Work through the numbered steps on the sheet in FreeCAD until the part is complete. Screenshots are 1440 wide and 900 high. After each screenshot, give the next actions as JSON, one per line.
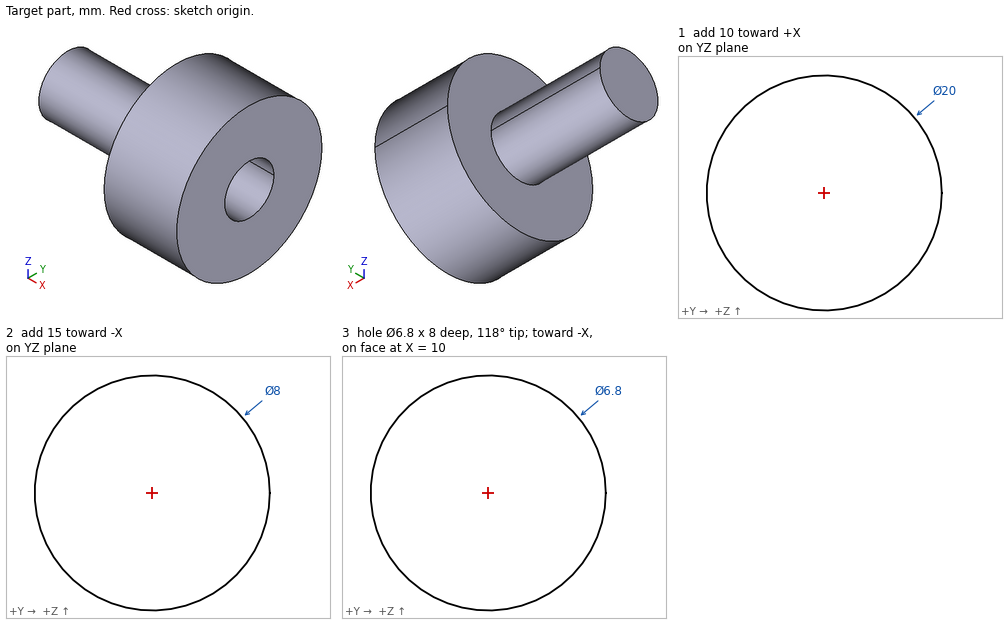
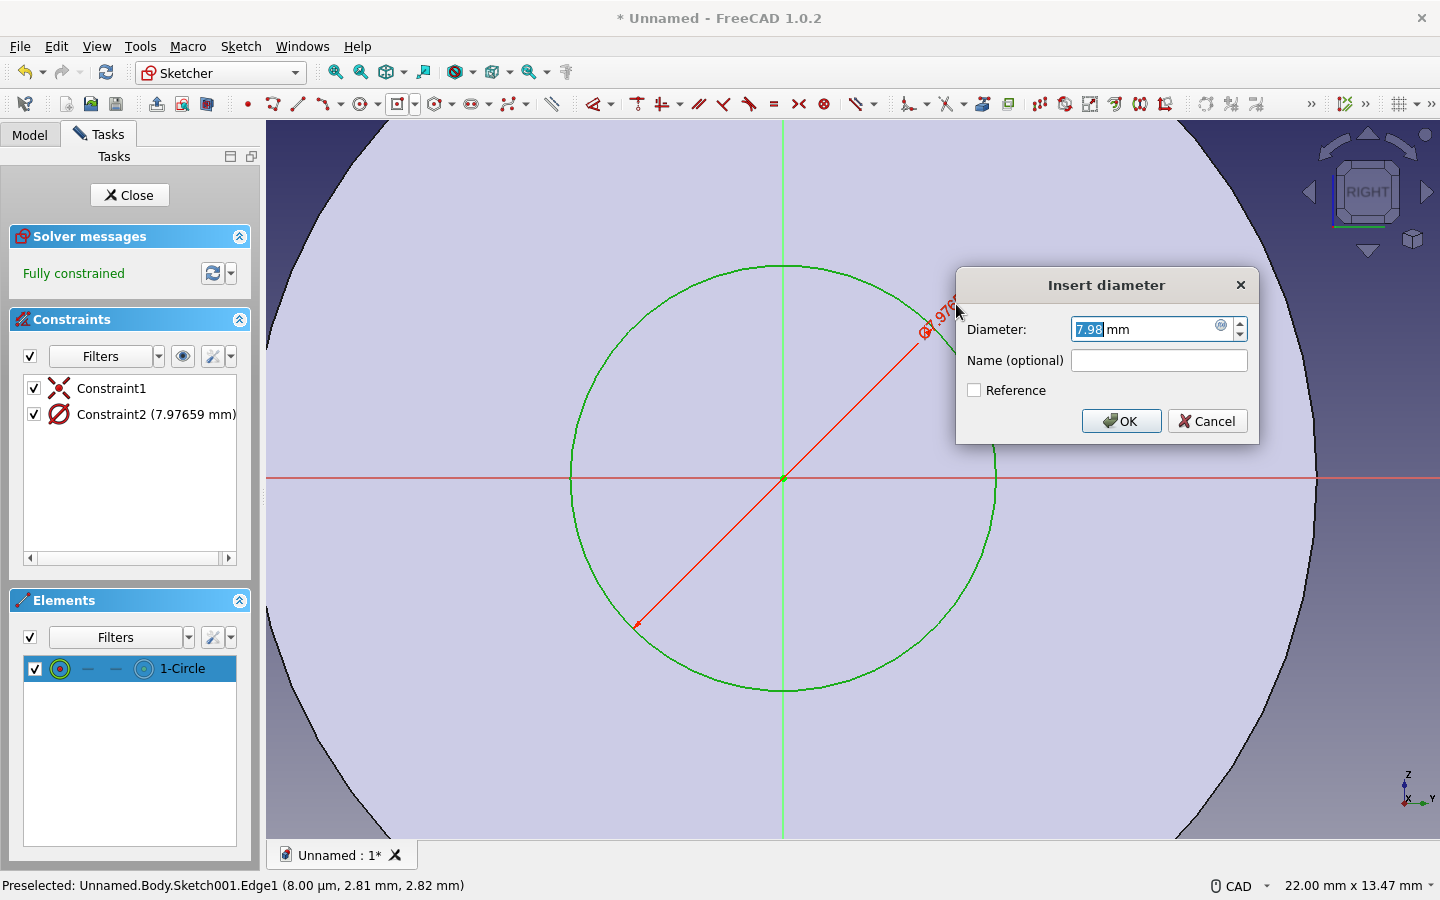
{"action": "type", "text": "8"}
{"action": "key", "text": "Return"}
{"action": "key", "text": "Escape"}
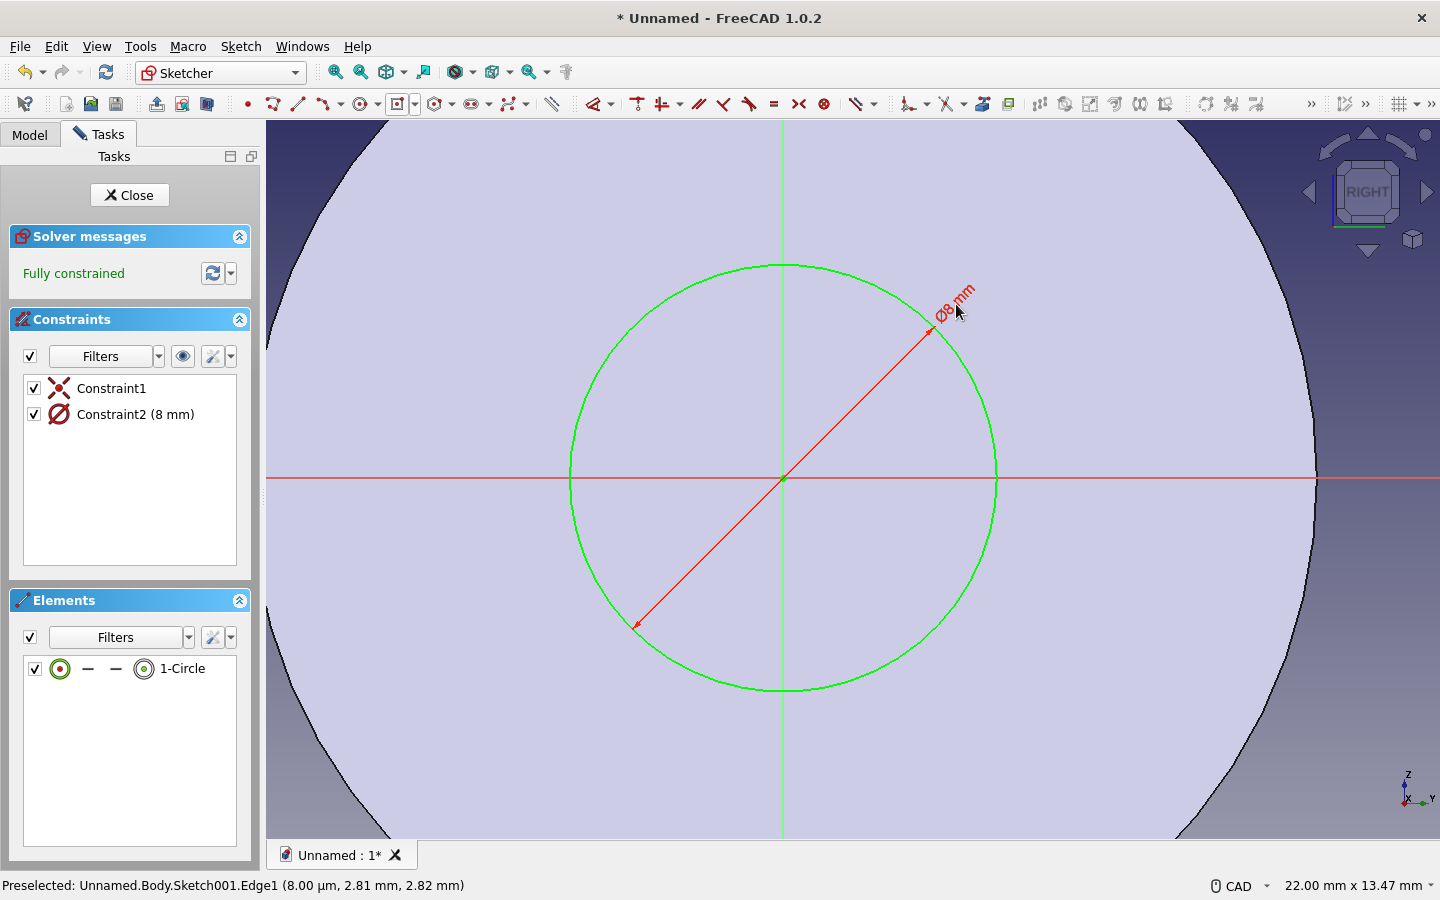
{"action": "left_click", "coordinate": [130, 195]}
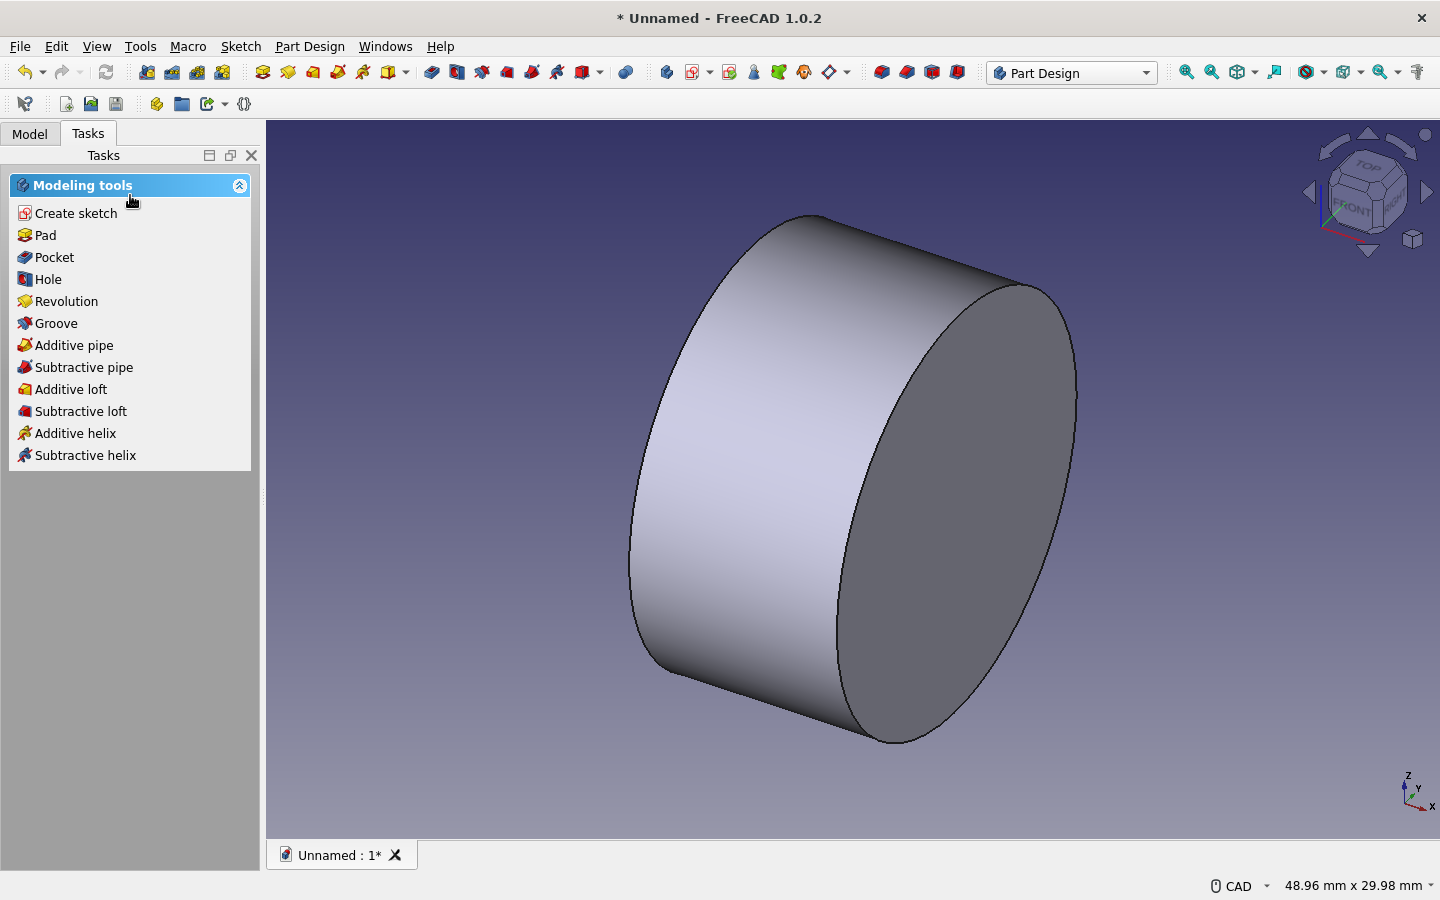
{"action": "left_click", "coordinate": [263, 72]}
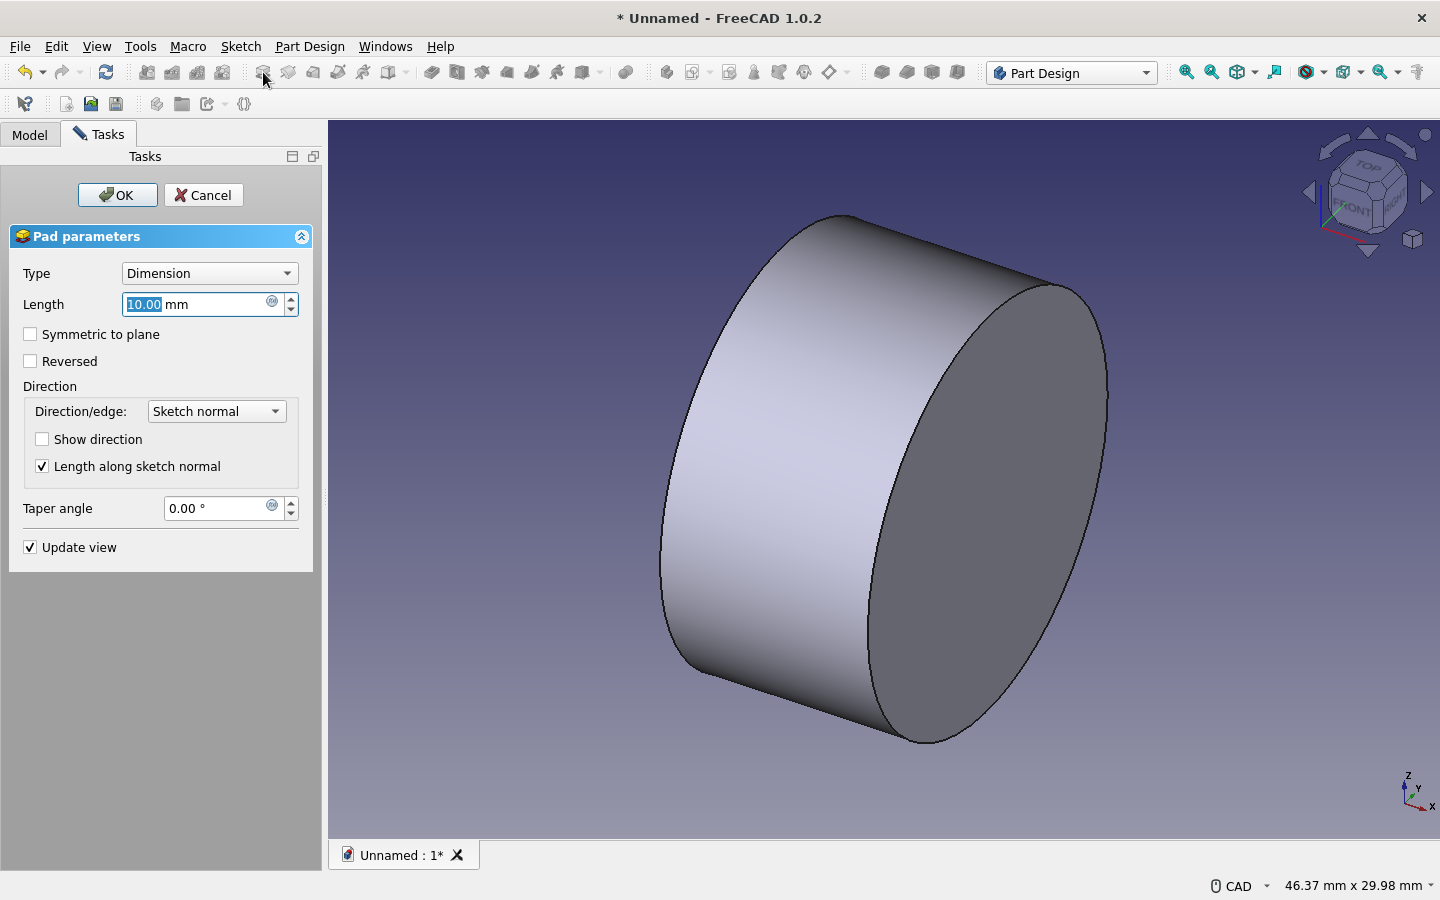
{"action": "type", "text": "15"}
{"action": "key", "text": "Tab"}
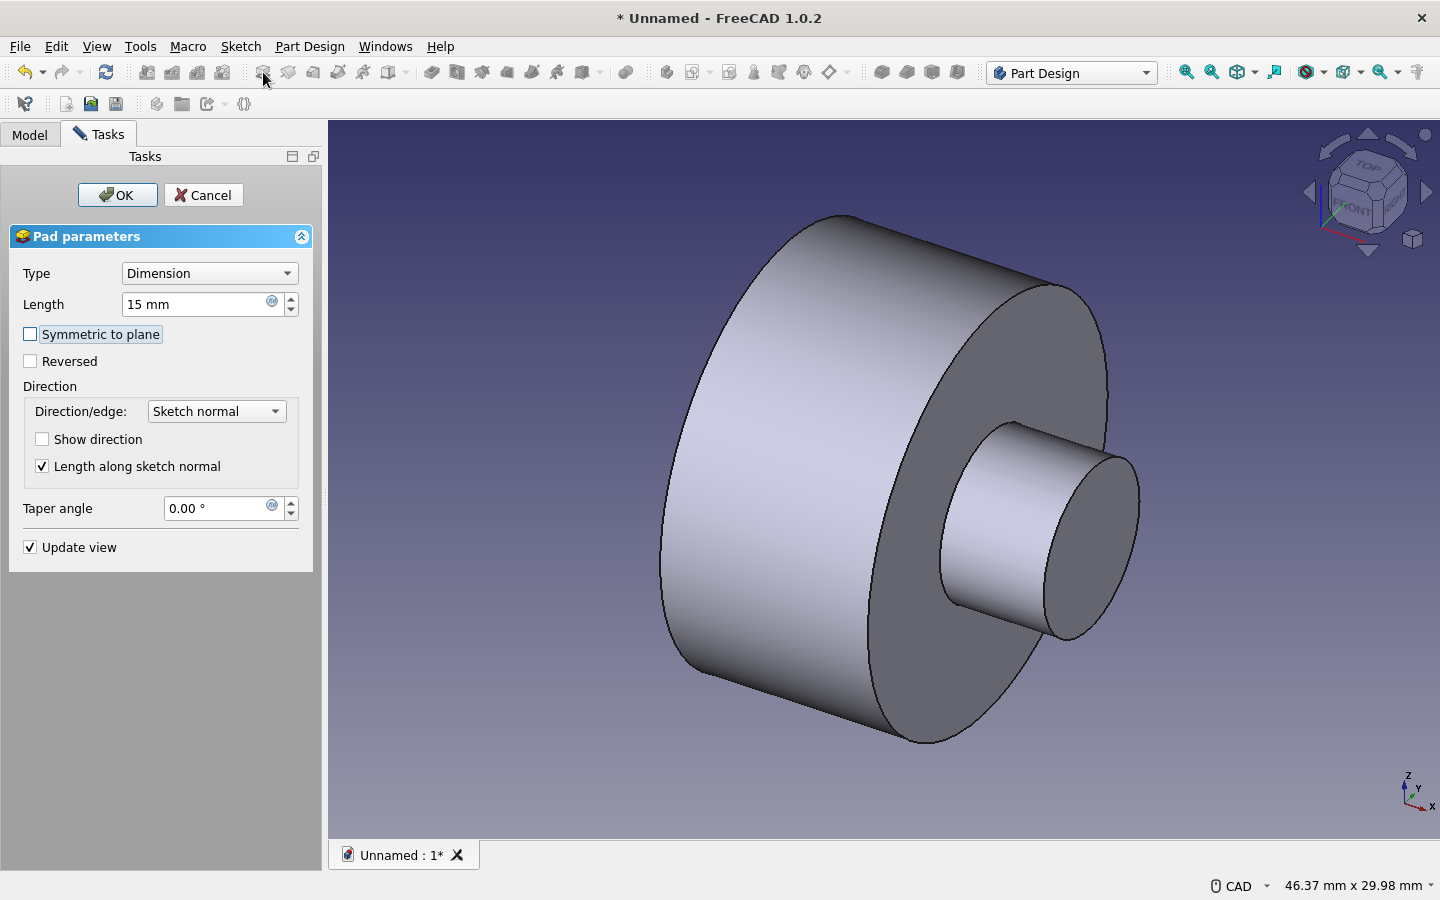
{"action": "left_click", "coordinate": [31, 361]}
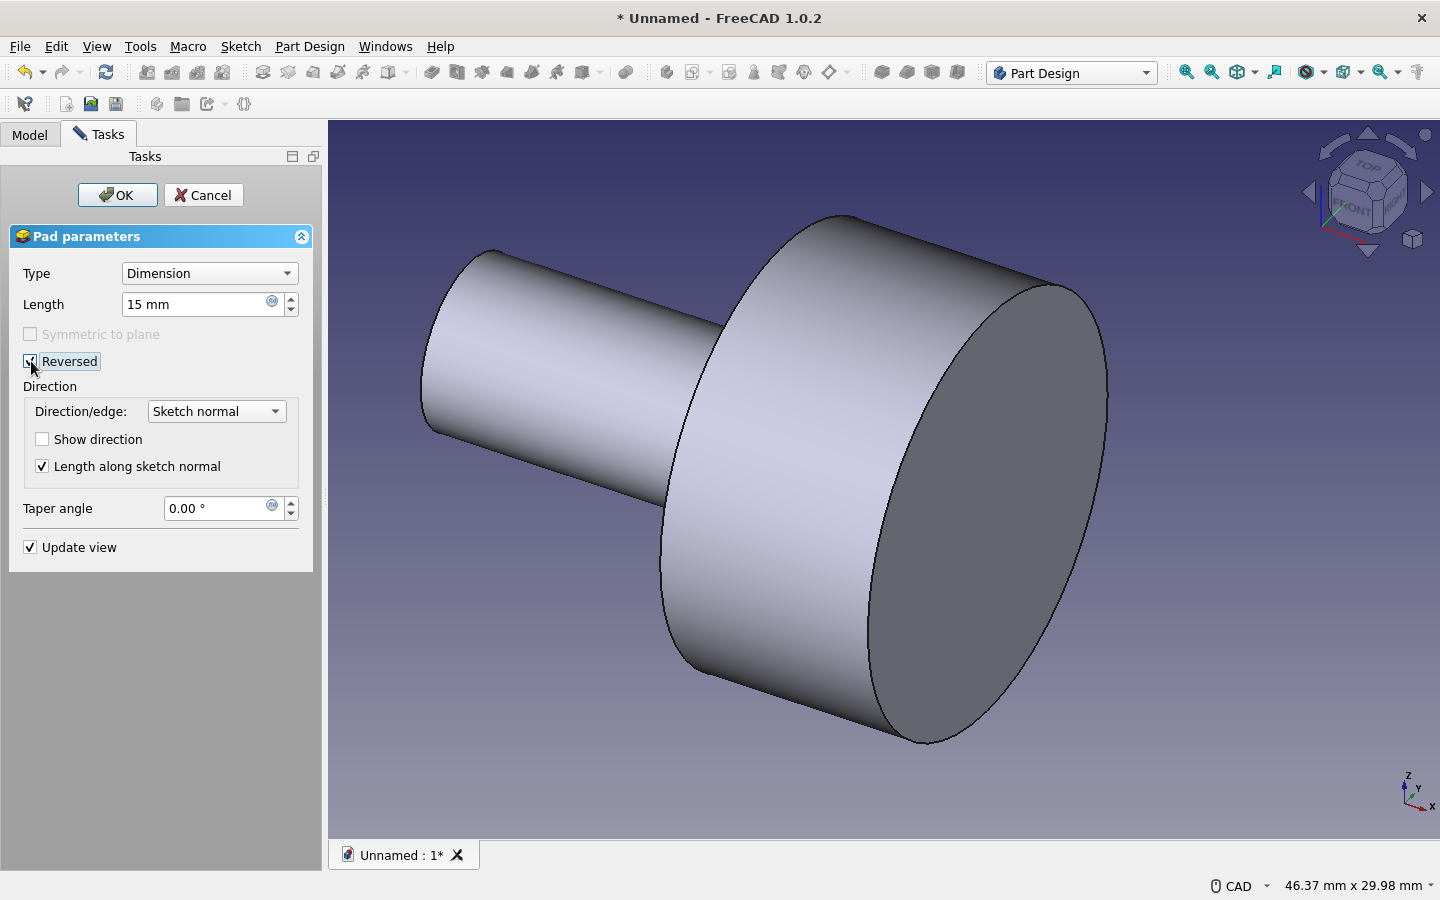
{"action": "left_click", "coordinate": [118, 195]}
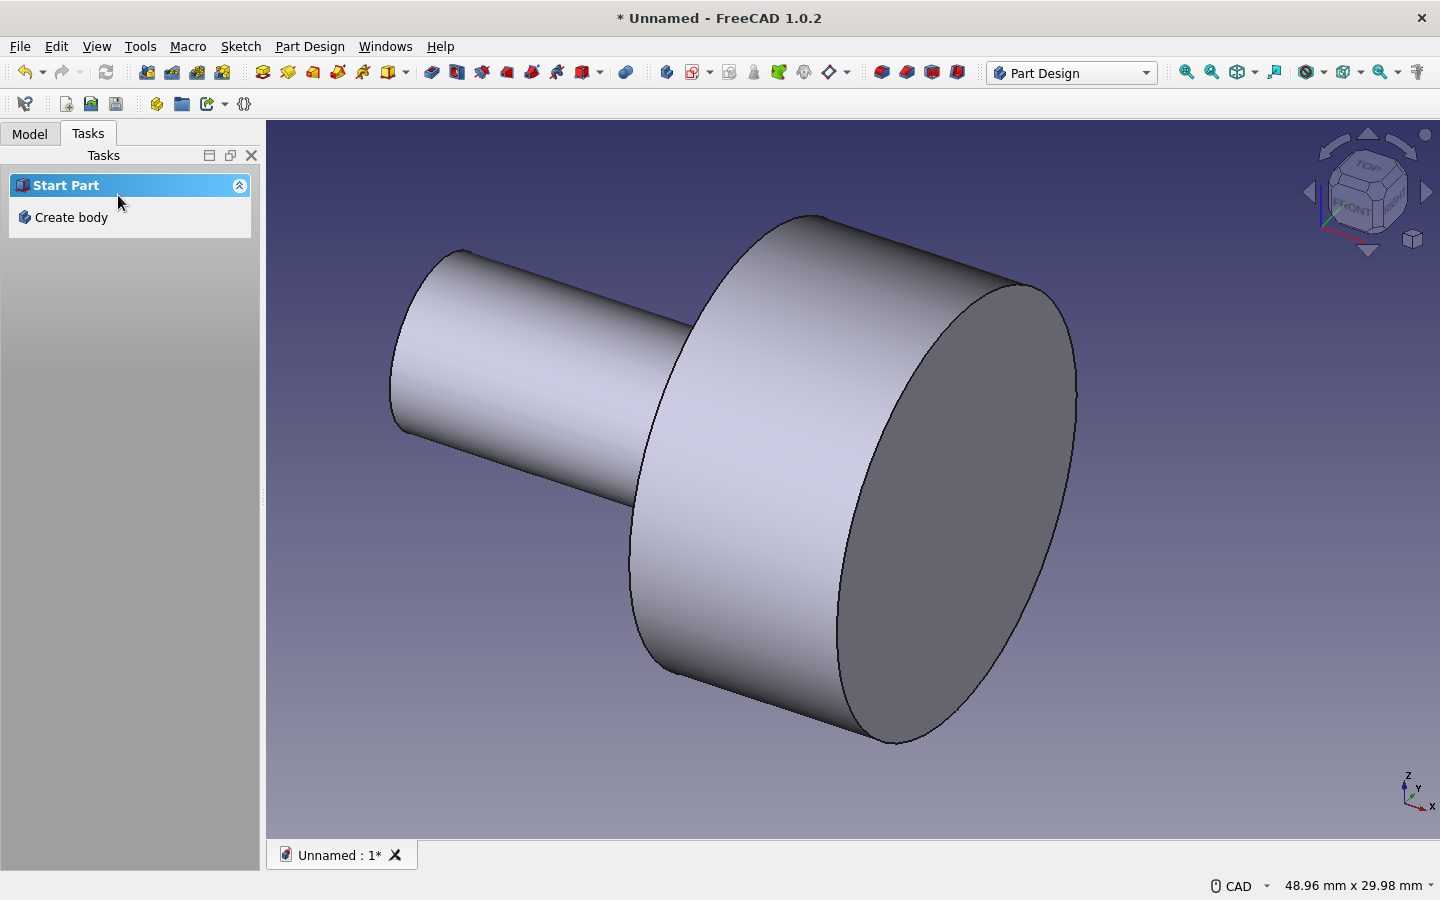
{"action": "left_click", "coordinate": [1187, 72]}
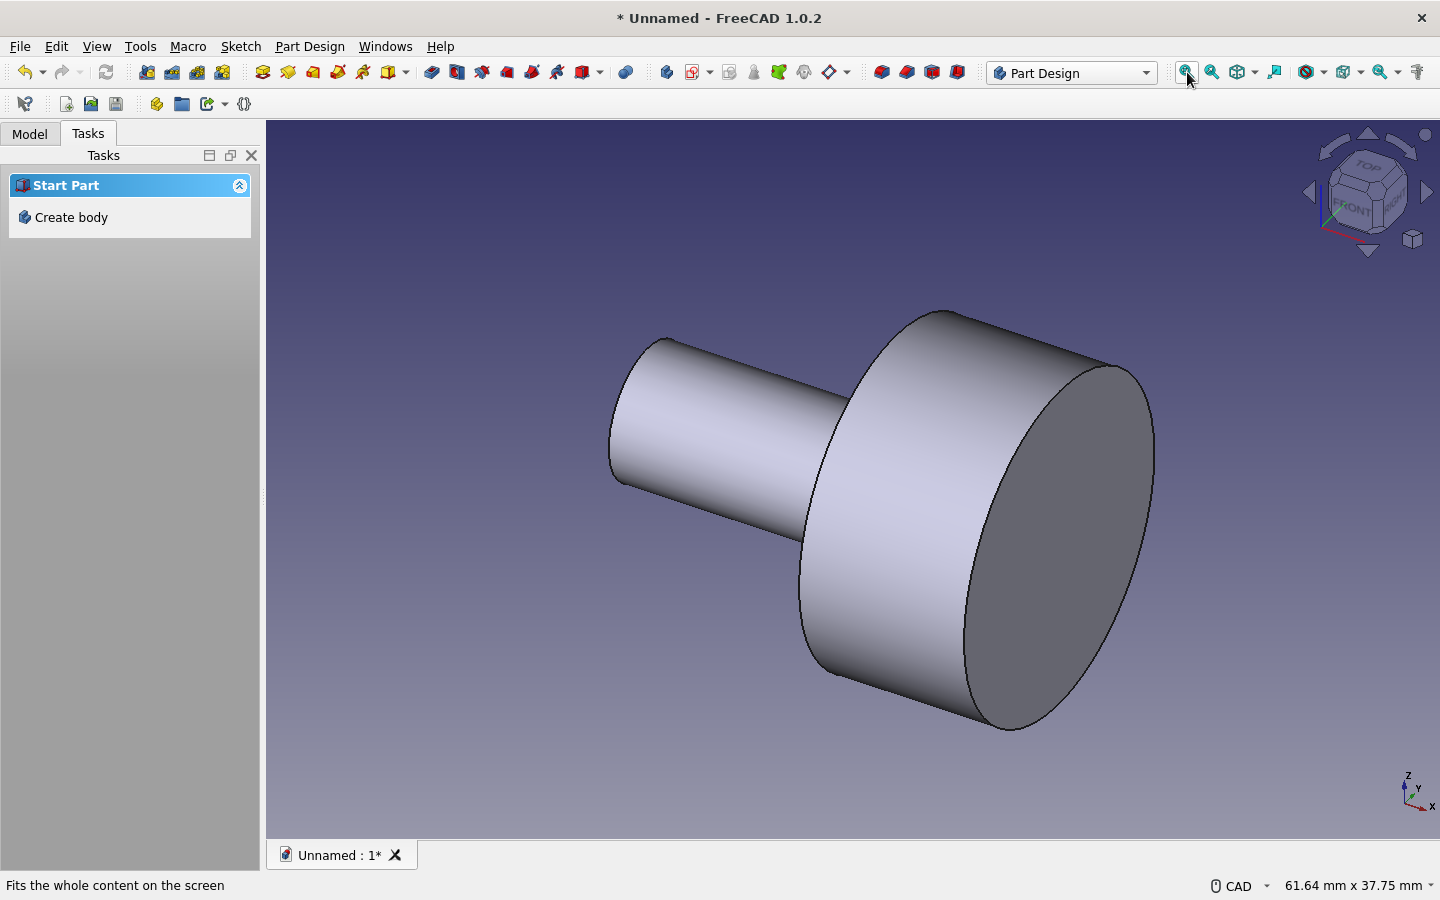
{"action": "left_click", "coordinate": [1059, 547]}